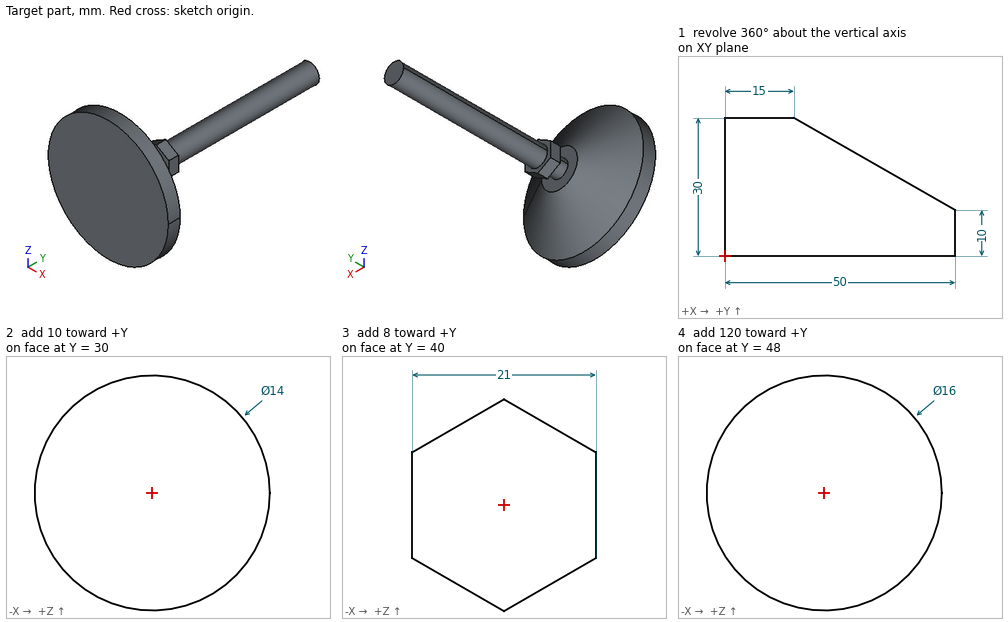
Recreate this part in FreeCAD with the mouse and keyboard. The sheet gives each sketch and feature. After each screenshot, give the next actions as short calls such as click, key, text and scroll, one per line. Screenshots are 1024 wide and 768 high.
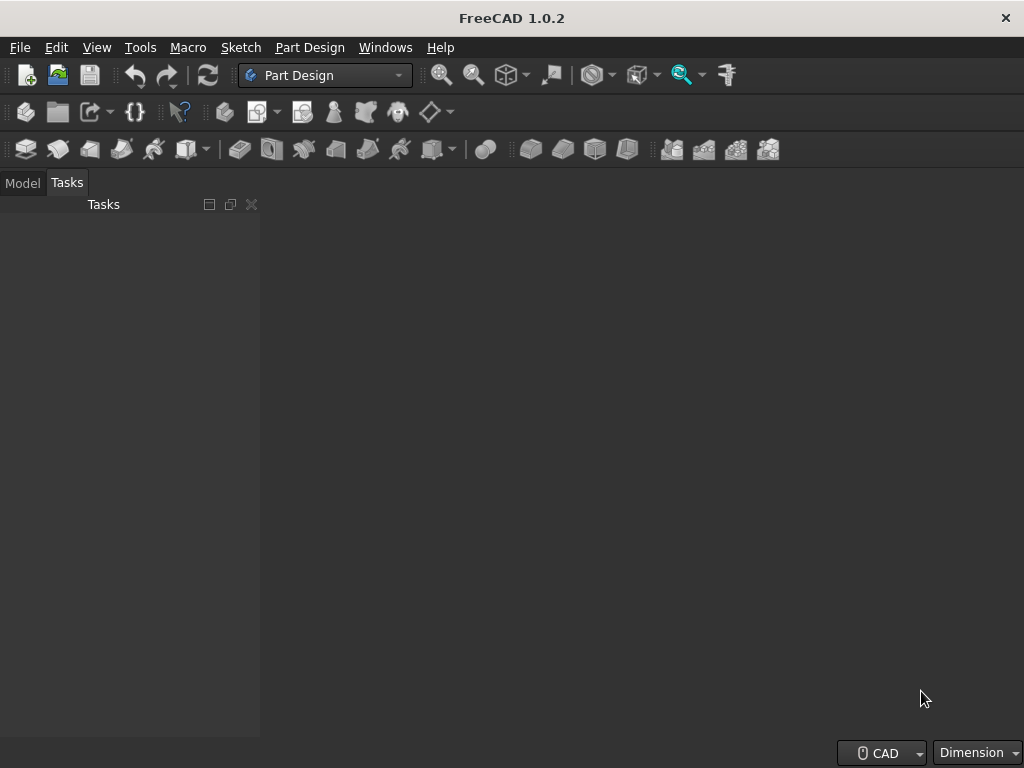
click(26, 76)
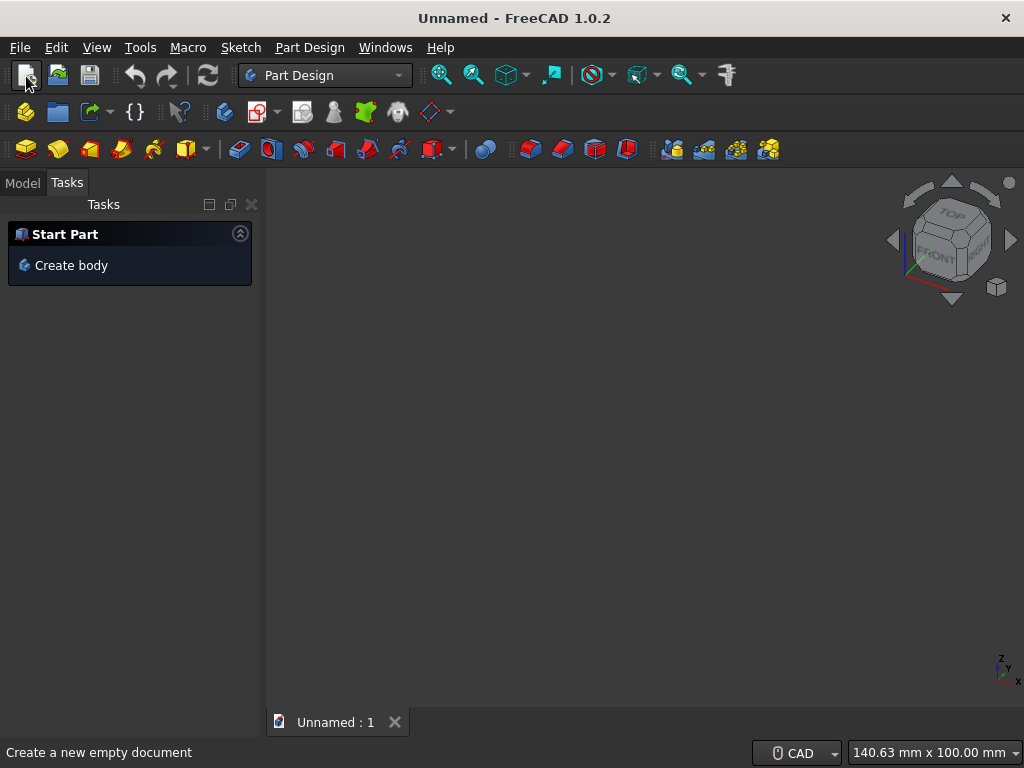
click(258, 112)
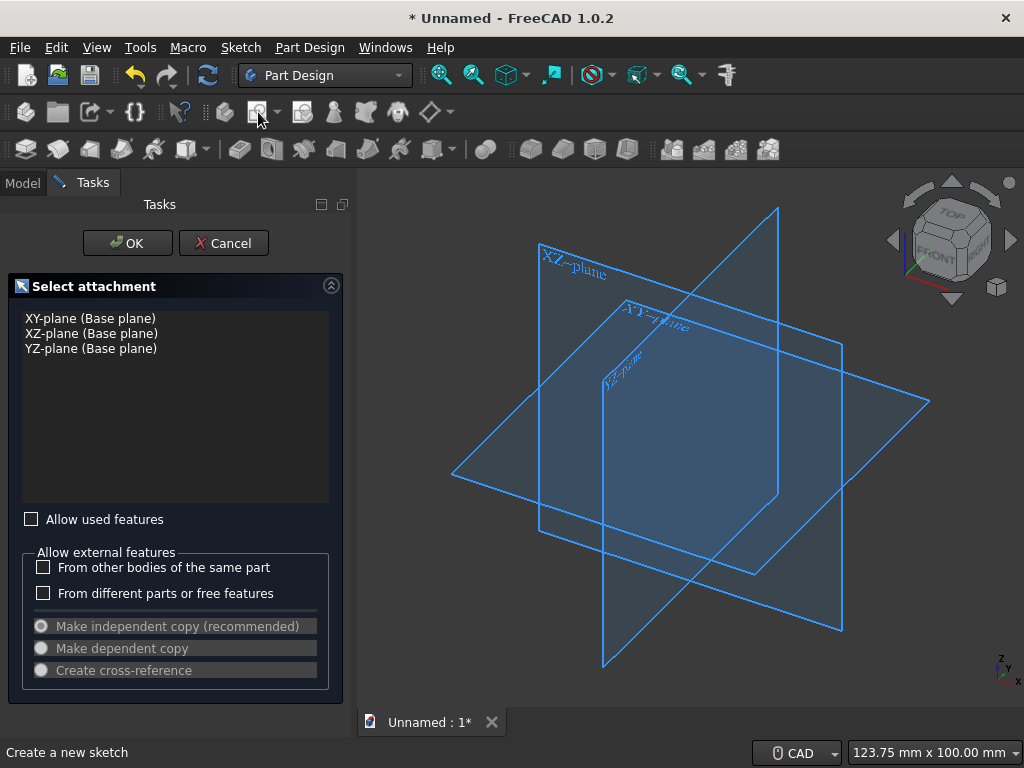
click(82, 318)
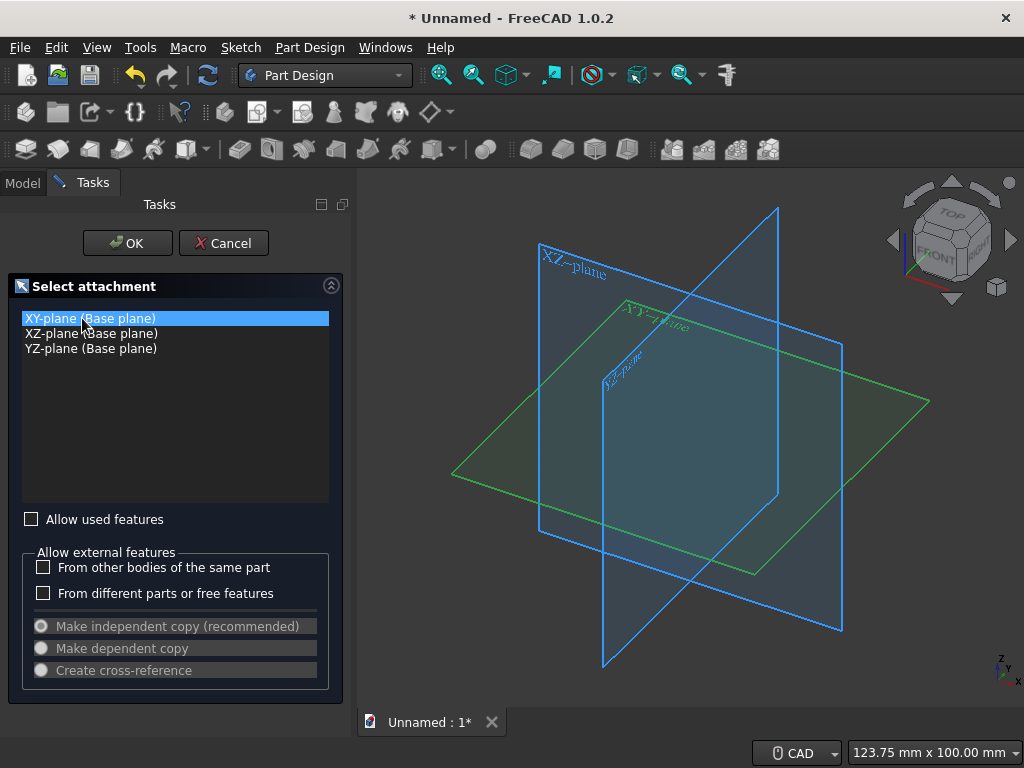
click(128, 243)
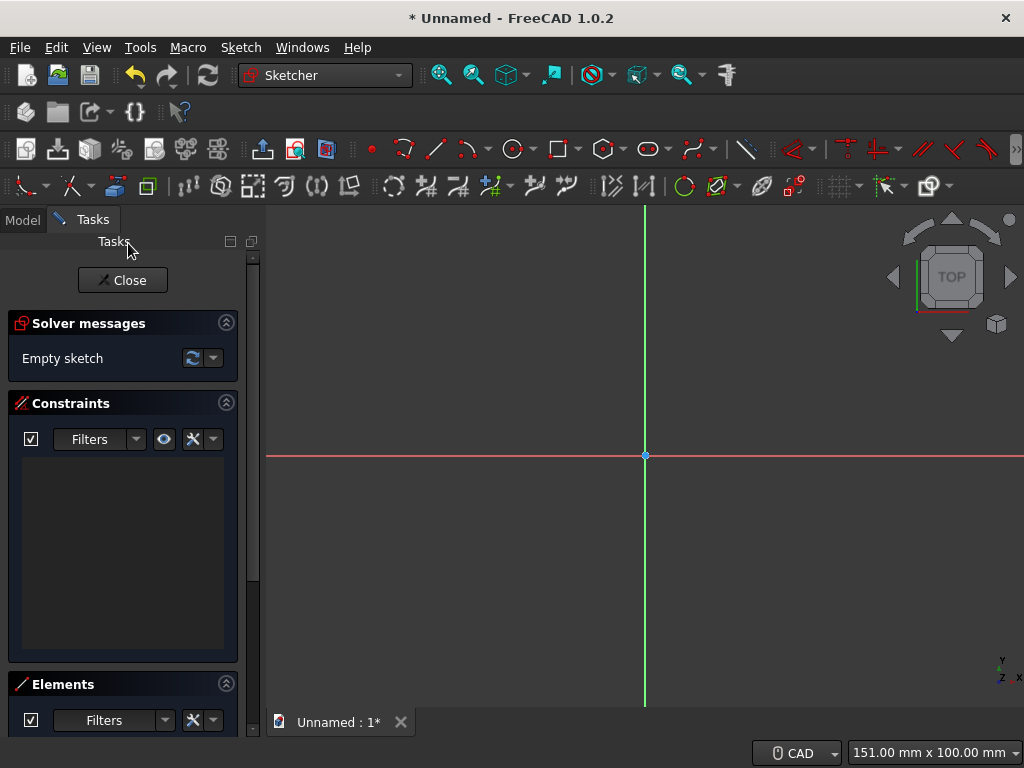
scroll(294, 679, down, 1)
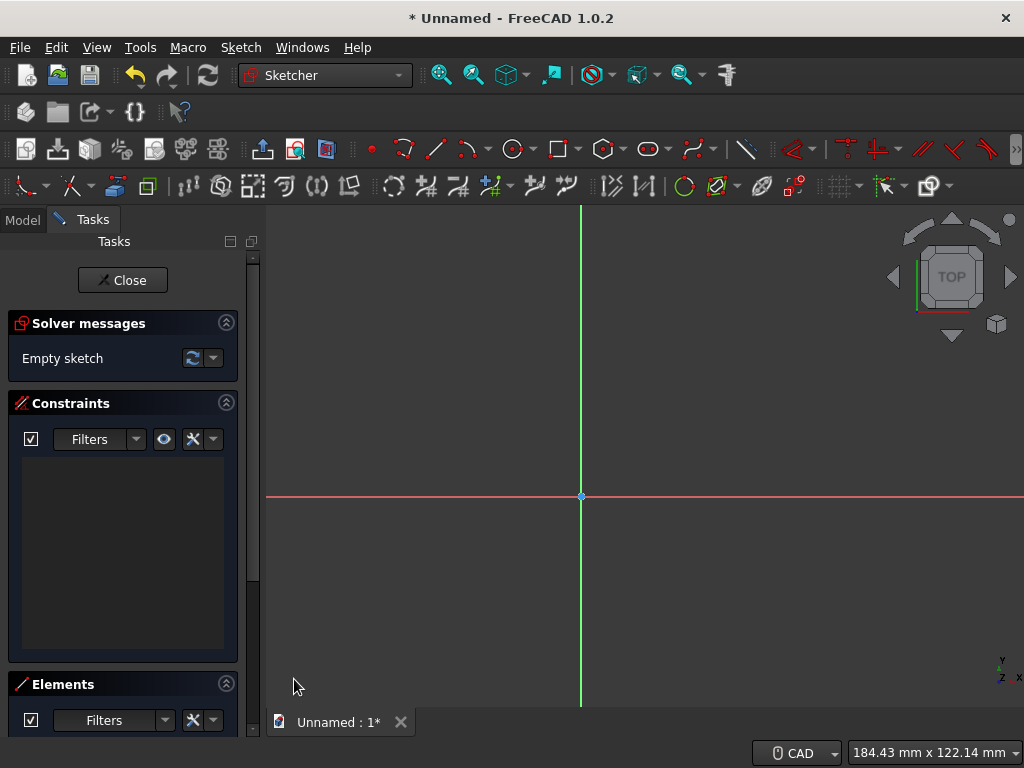
scroll(815, 409, up, 3)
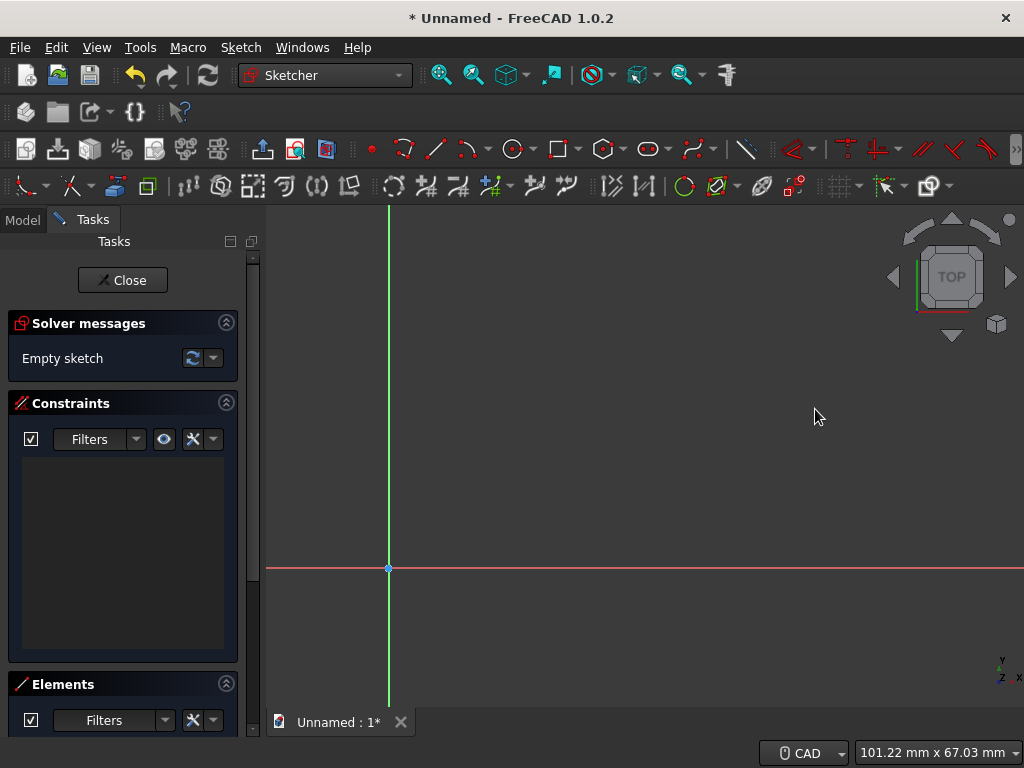
click(404, 150)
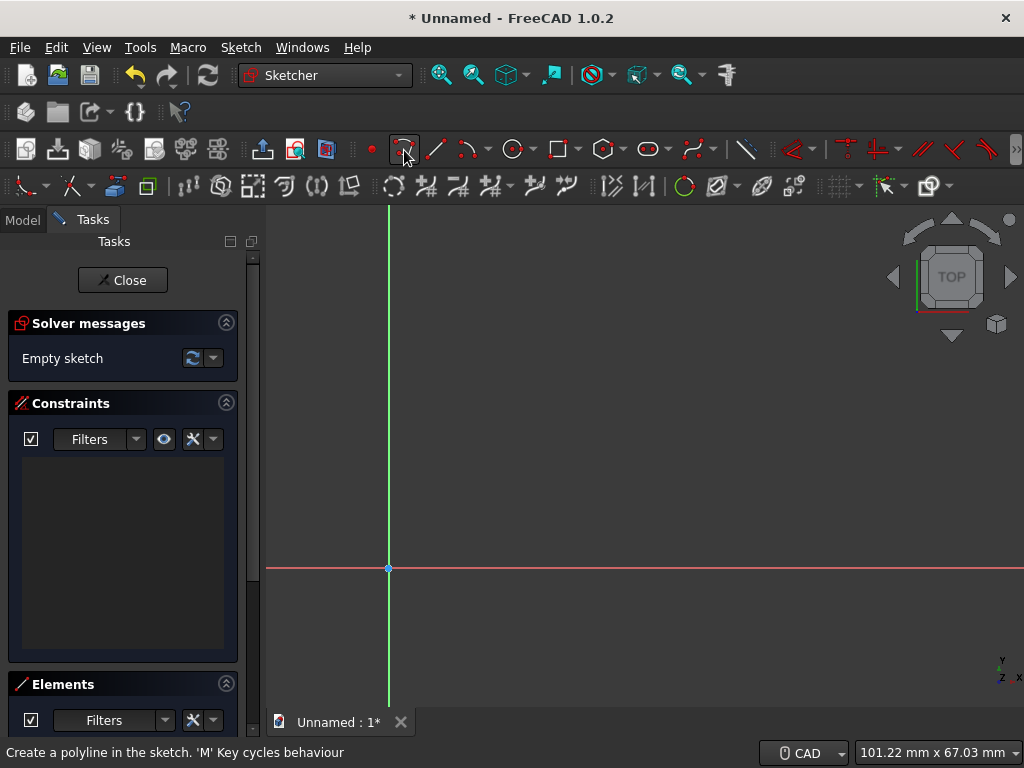
click(389, 568)
click(763, 559)
click(763, 493)
click(501, 344)
click(398, 344)
click(389, 568)
key(Escape)
key(Escape)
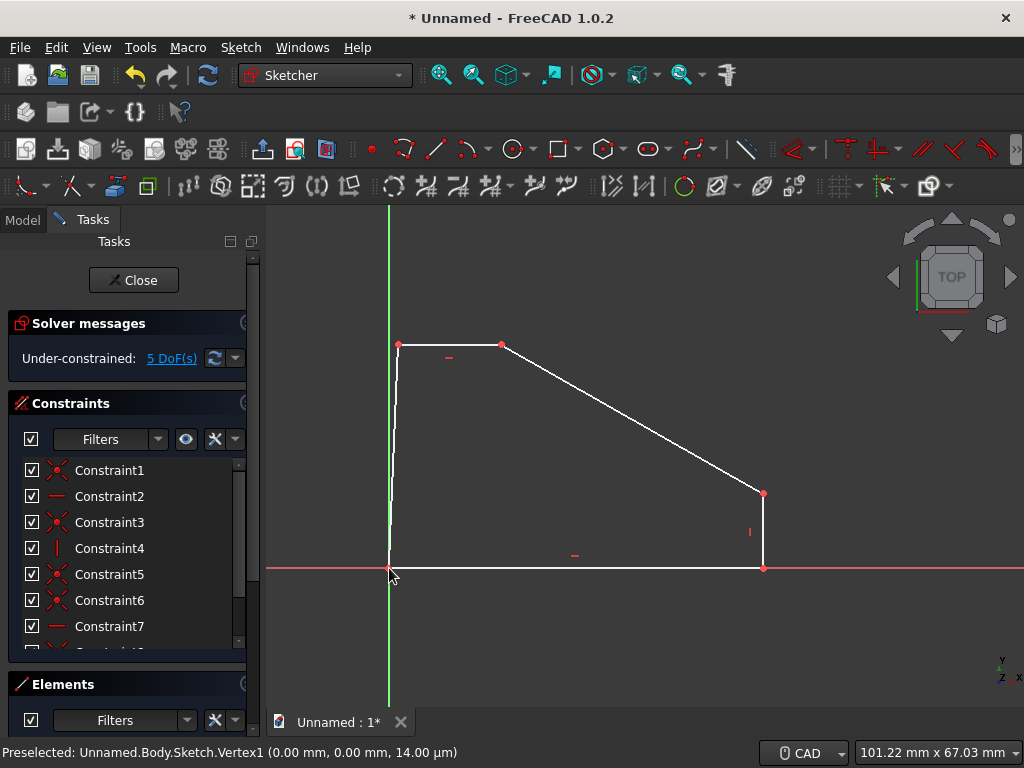
click(392, 501)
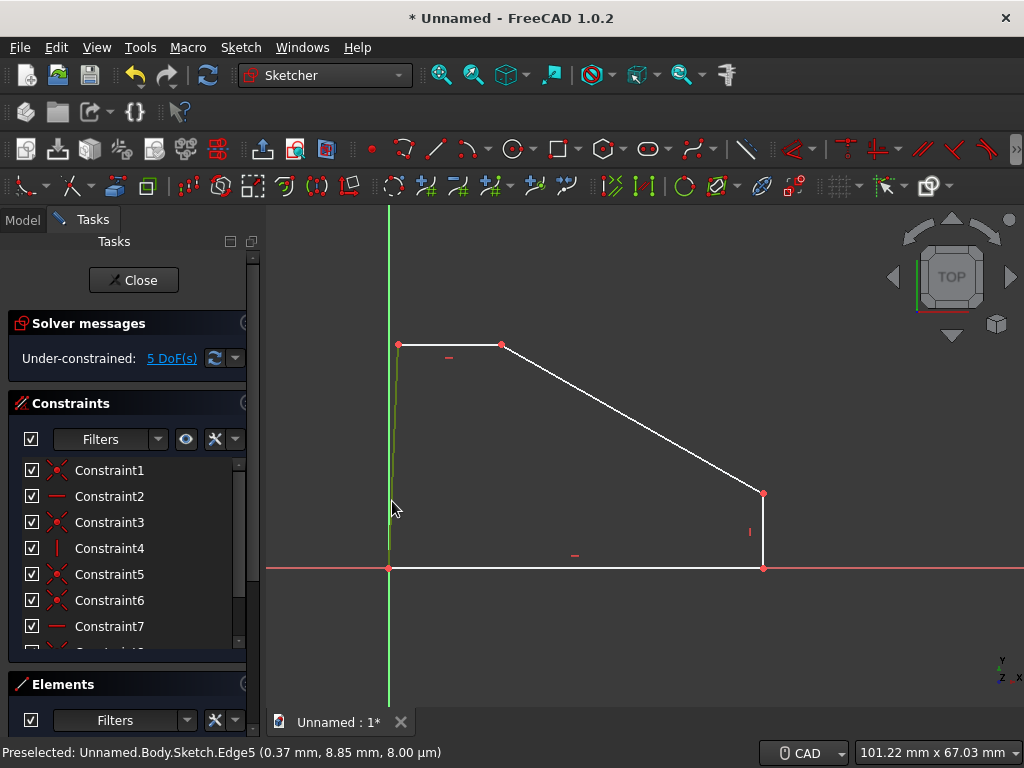
click(900, 150)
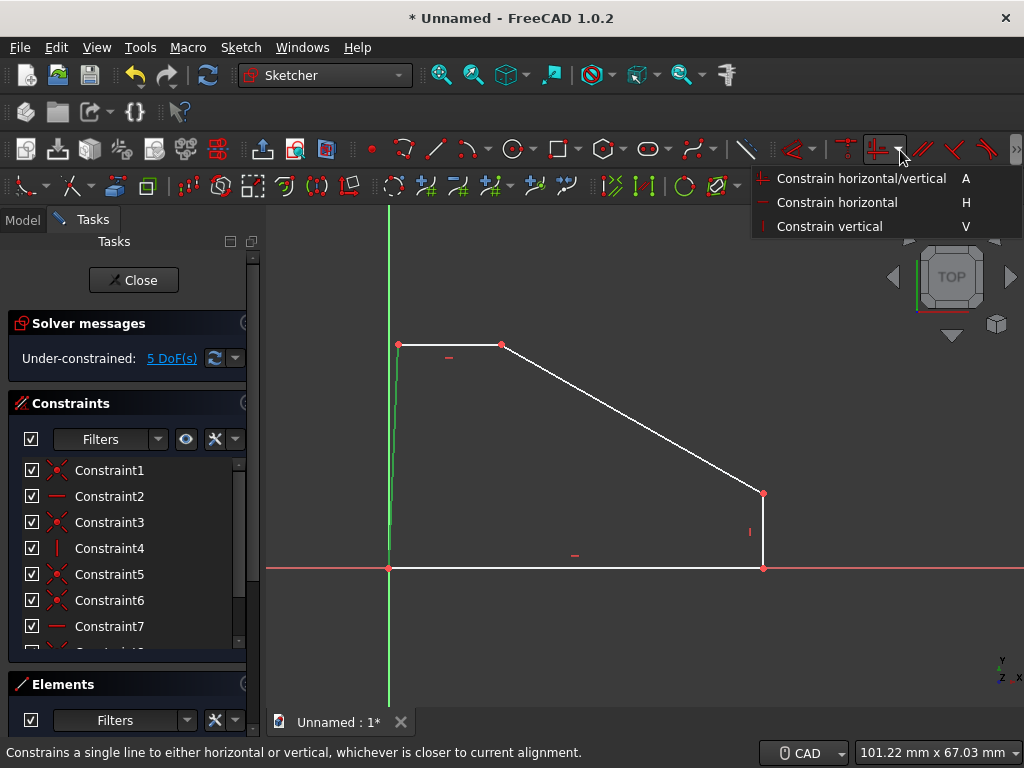
click(887, 226)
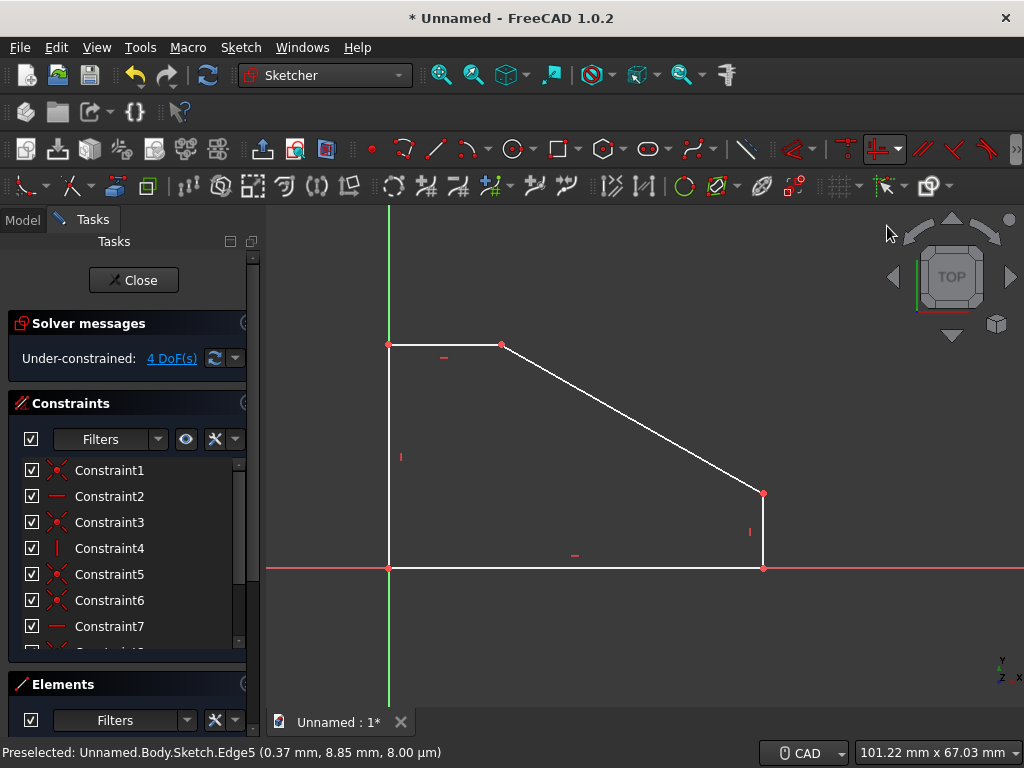
click(501, 568)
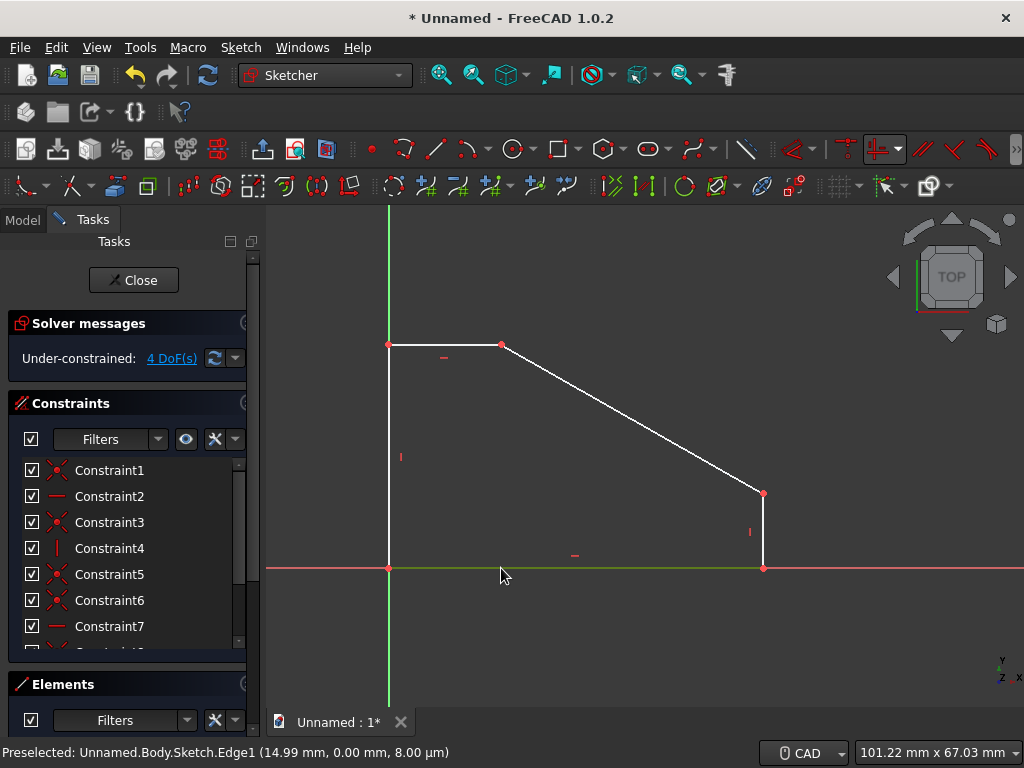
key(l)